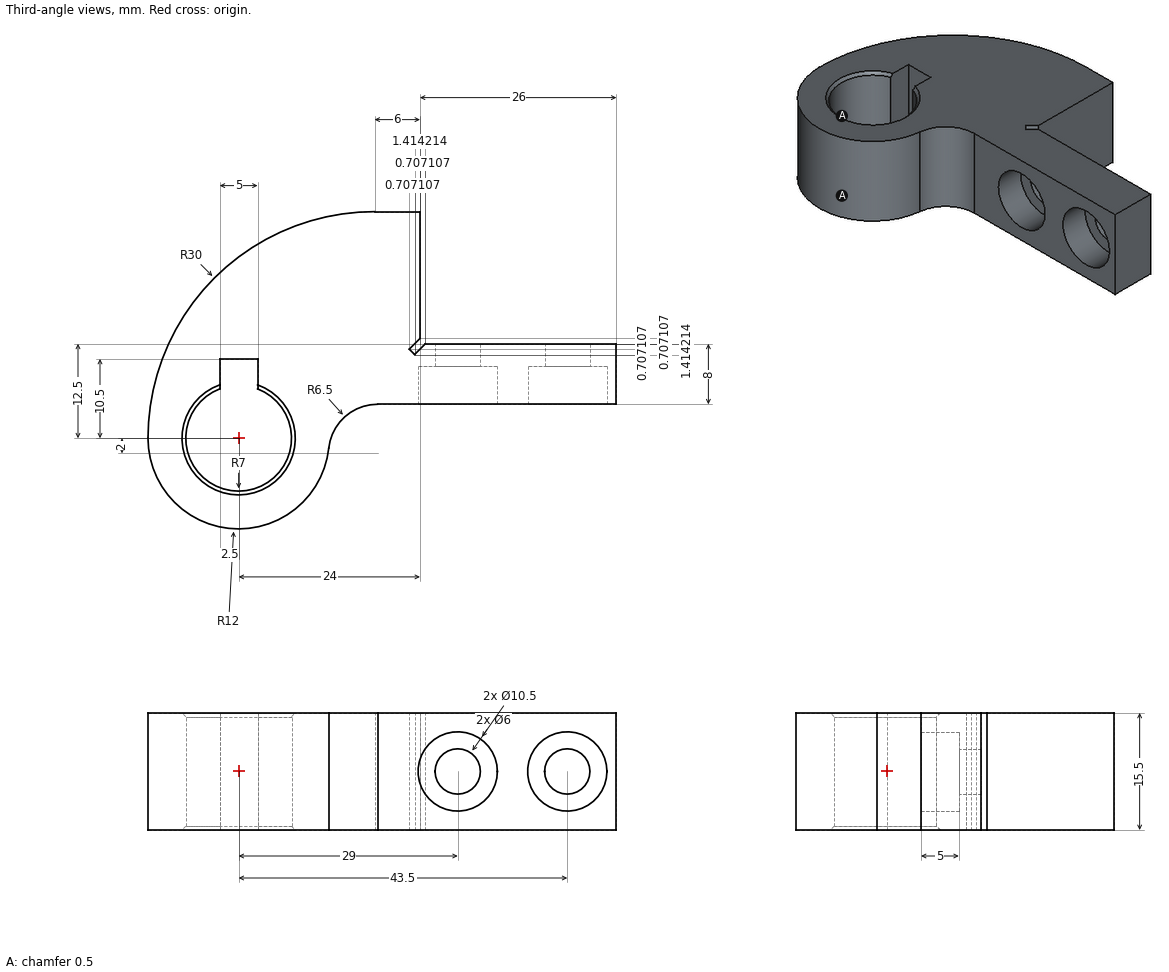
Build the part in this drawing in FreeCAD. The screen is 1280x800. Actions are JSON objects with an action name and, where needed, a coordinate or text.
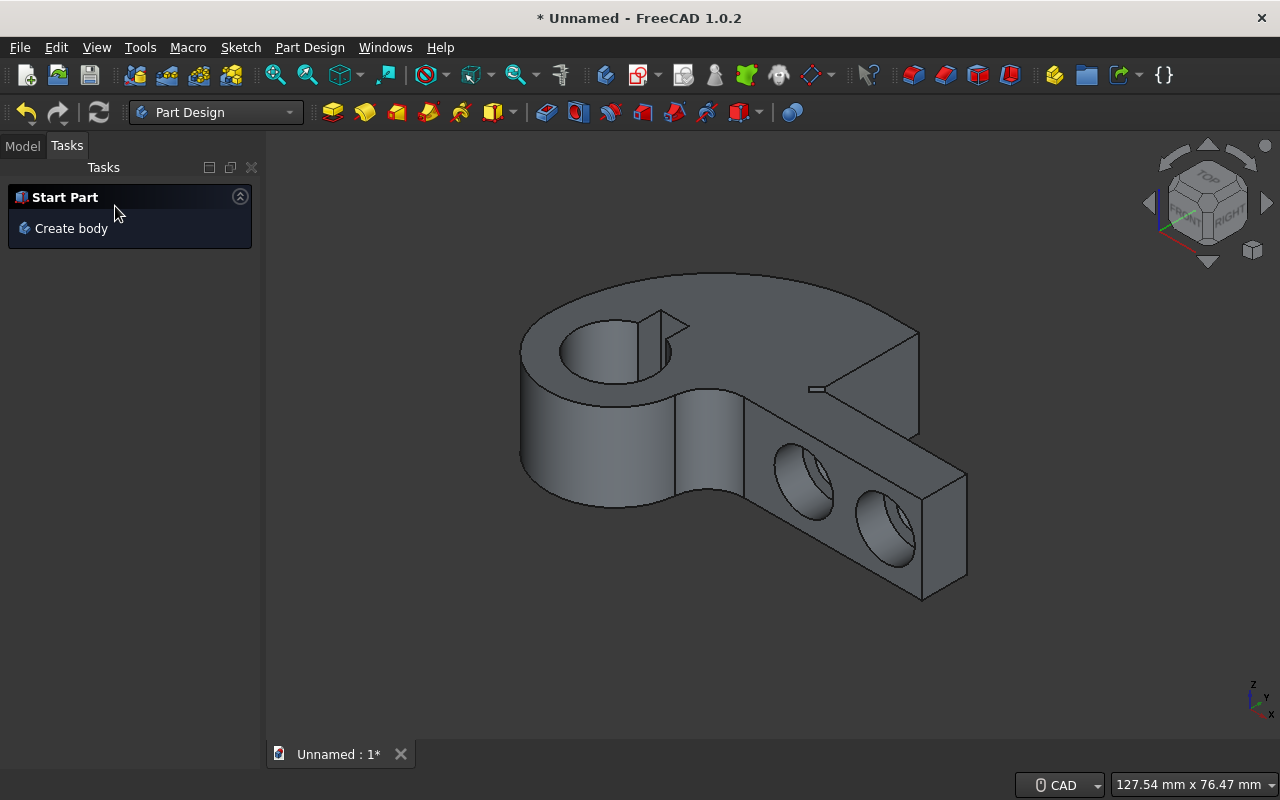
{"action": "left_click", "coordinate": [563, 341]}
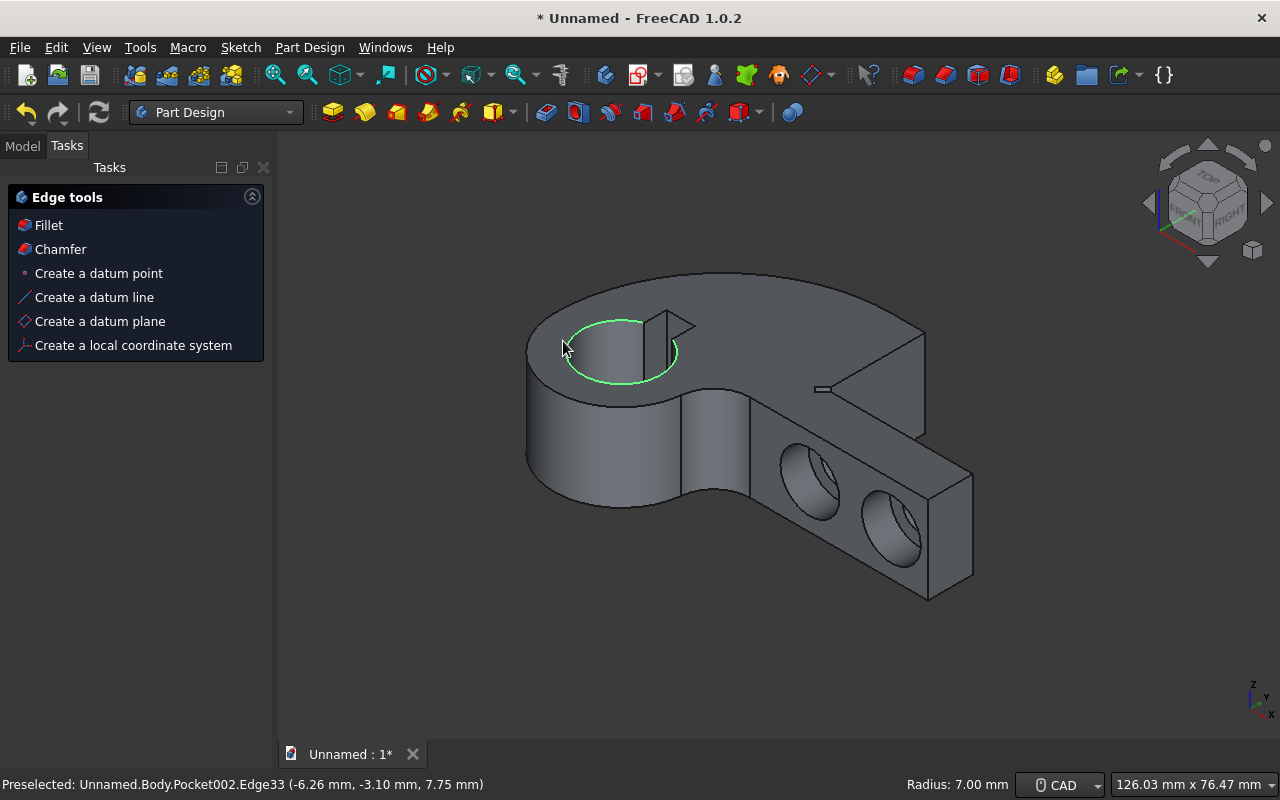
{"action": "key", "text": "2"}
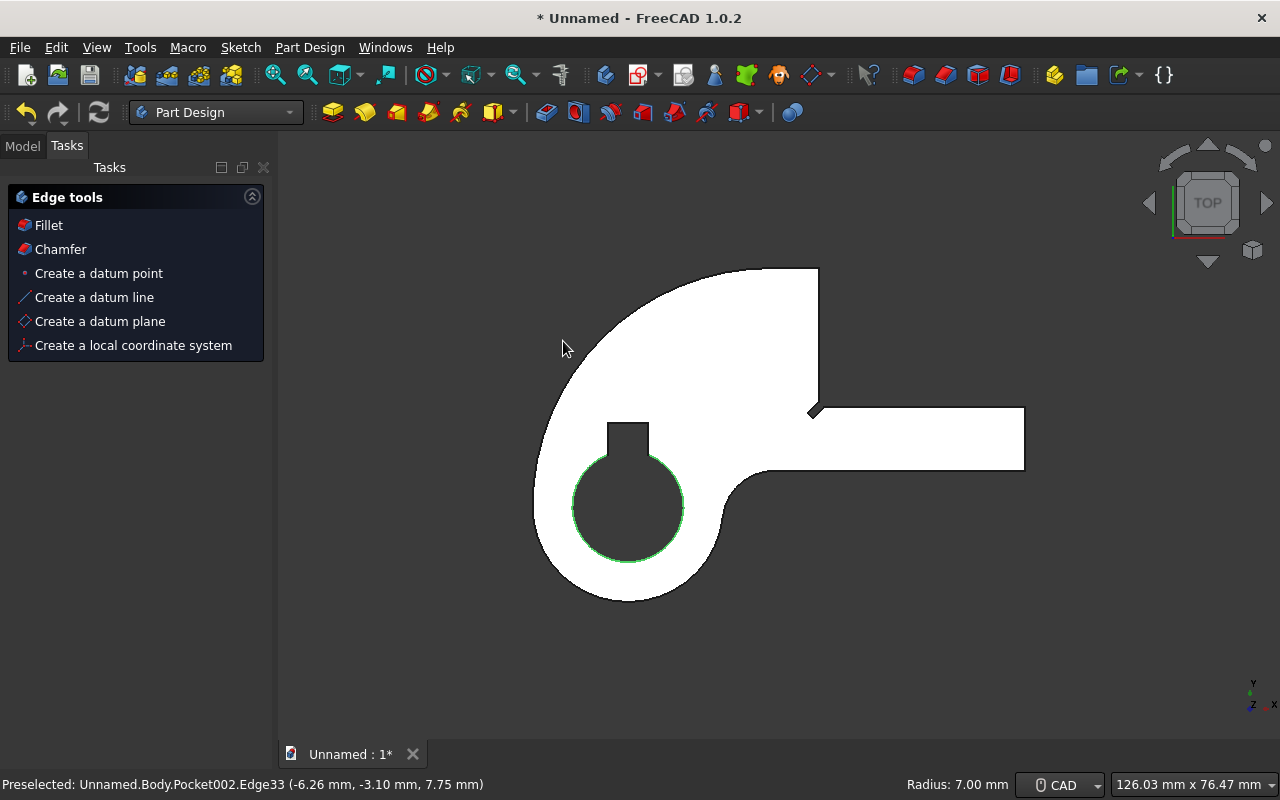
{"action": "key", "text": "0"}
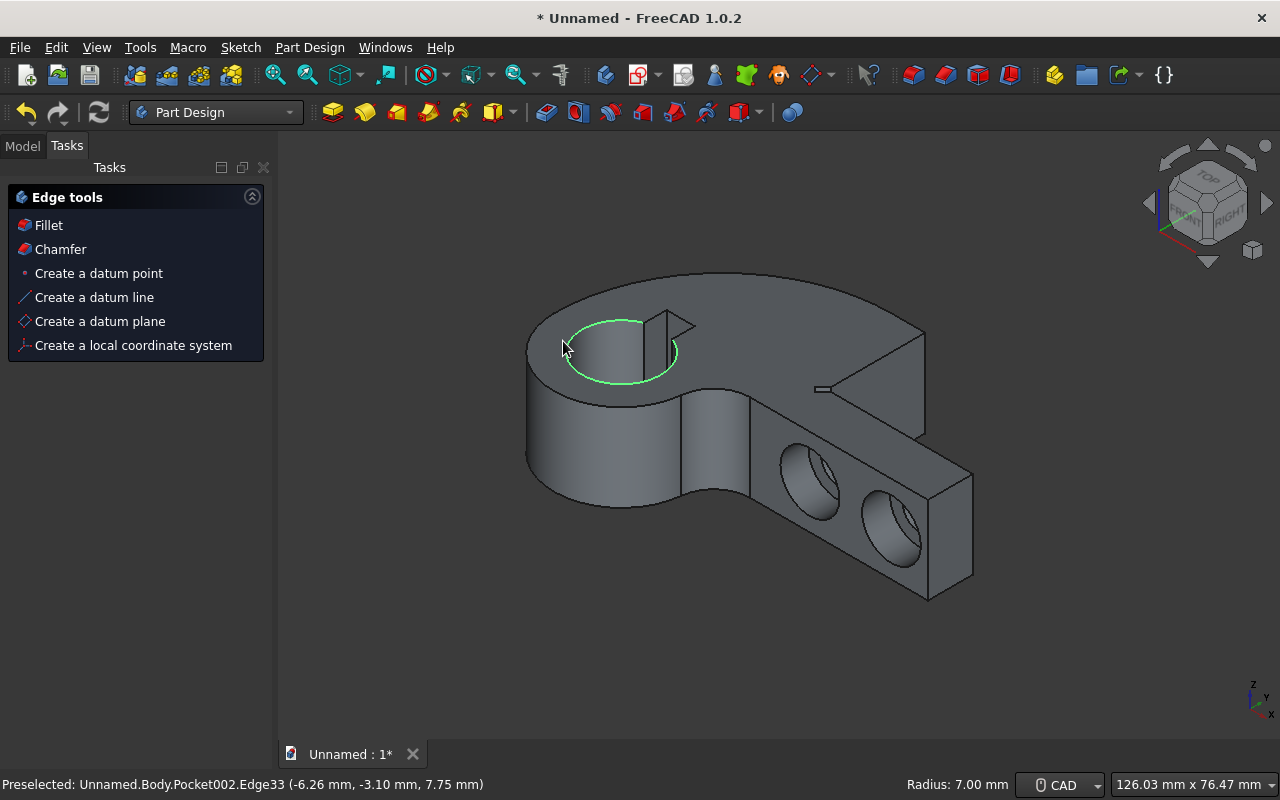
{"action": "key", "text": "1"}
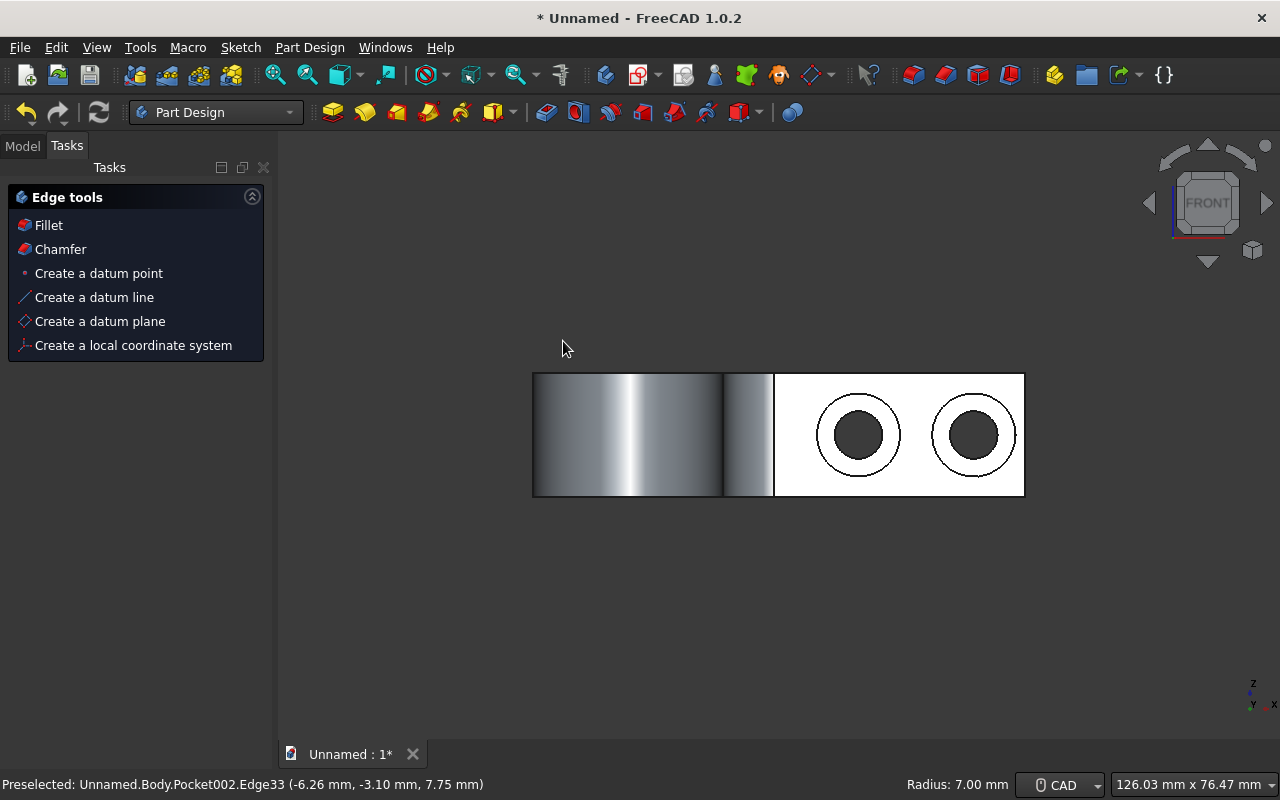
{"action": "key", "text": "3"}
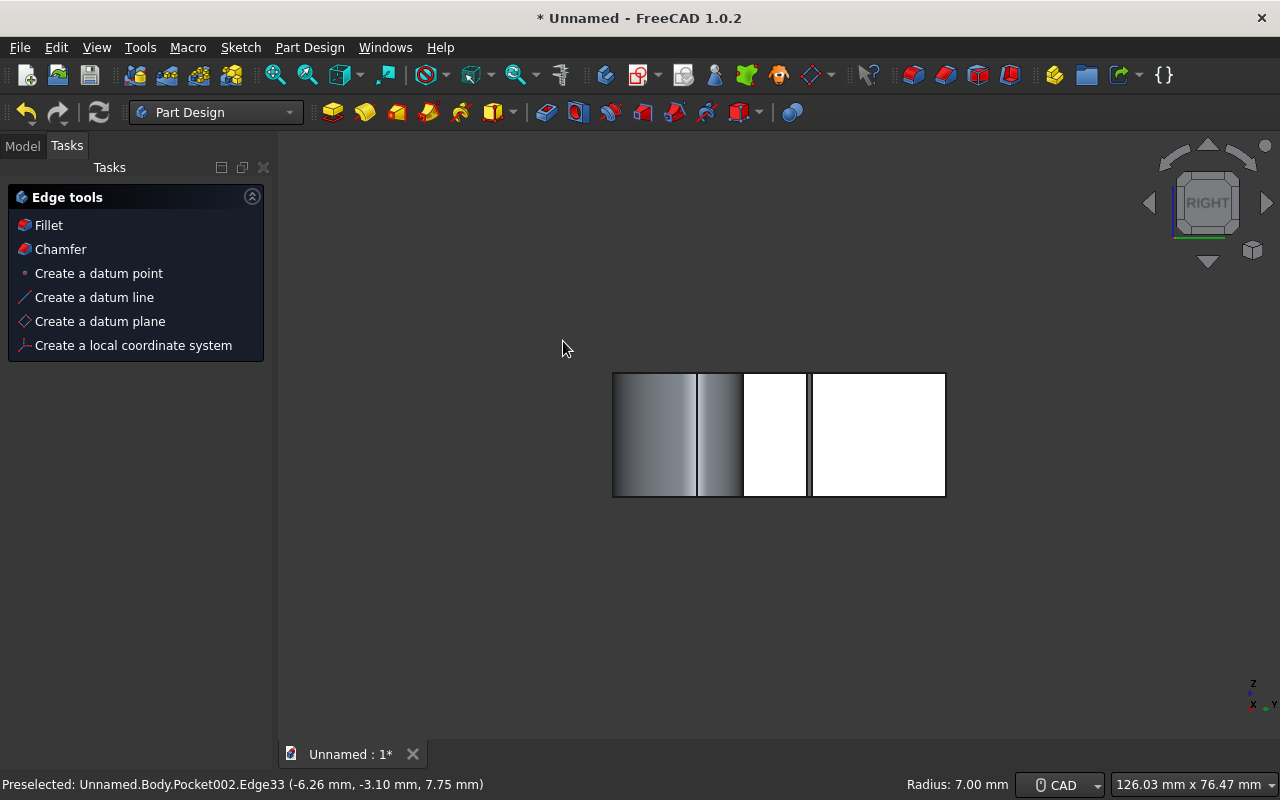
{"action": "left_click", "coordinate": [276, 76]}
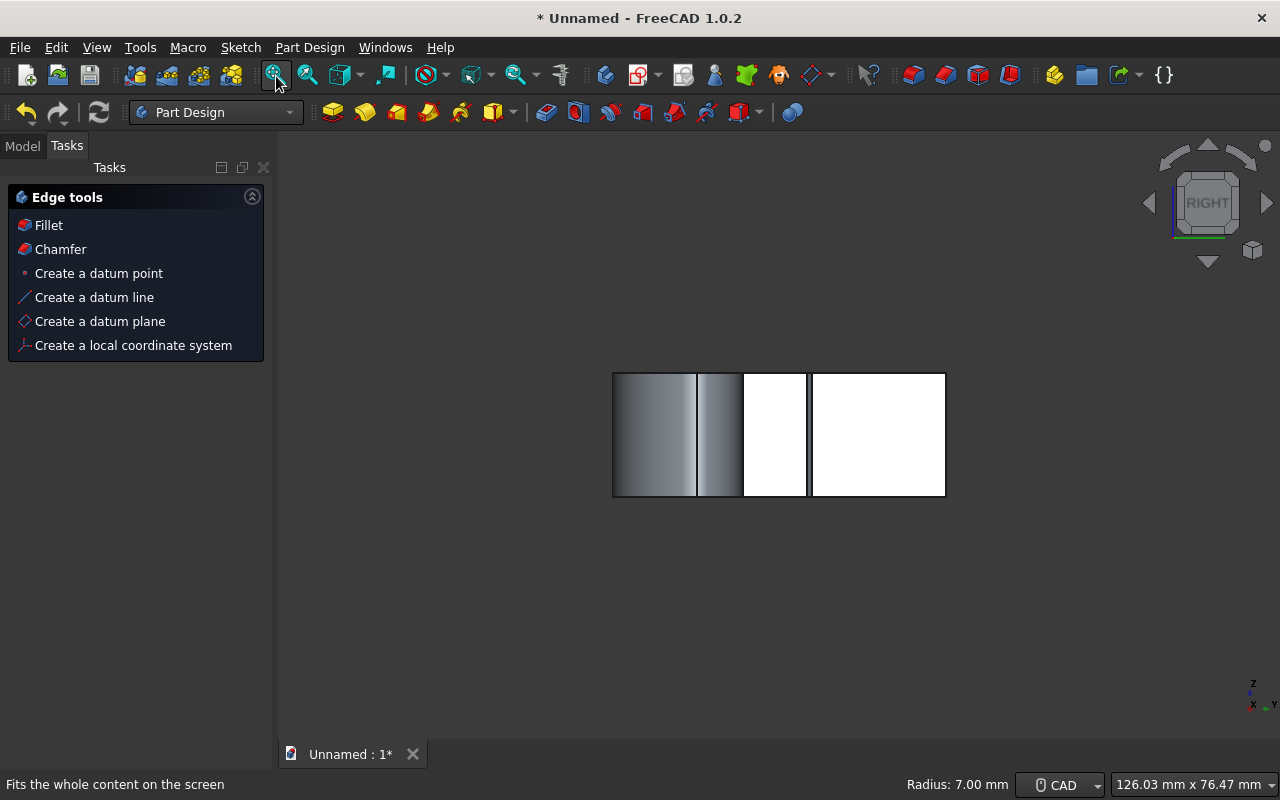
{"action": "key", "text": "5"}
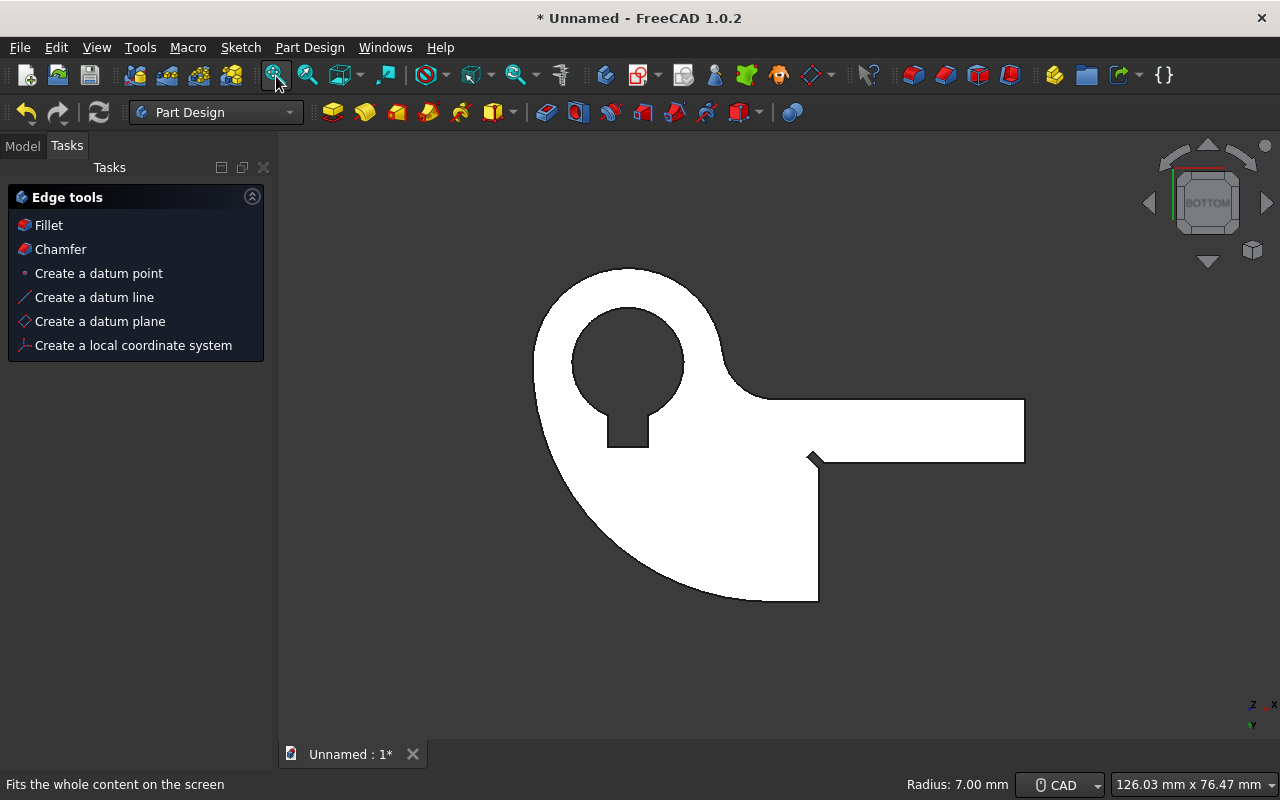
{"action": "left_click", "coordinate": [628, 307], "text": "ctrl"}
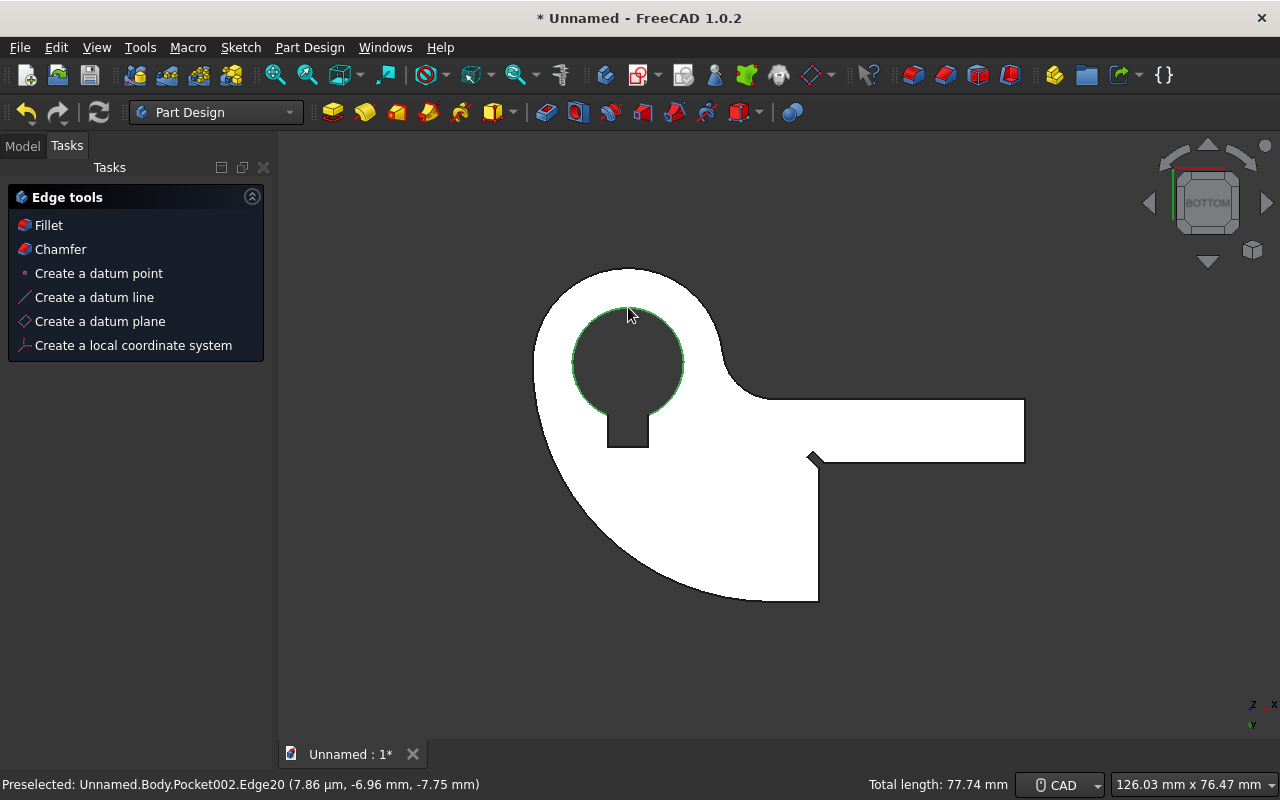
{"action": "left_click", "coordinate": [946, 76]}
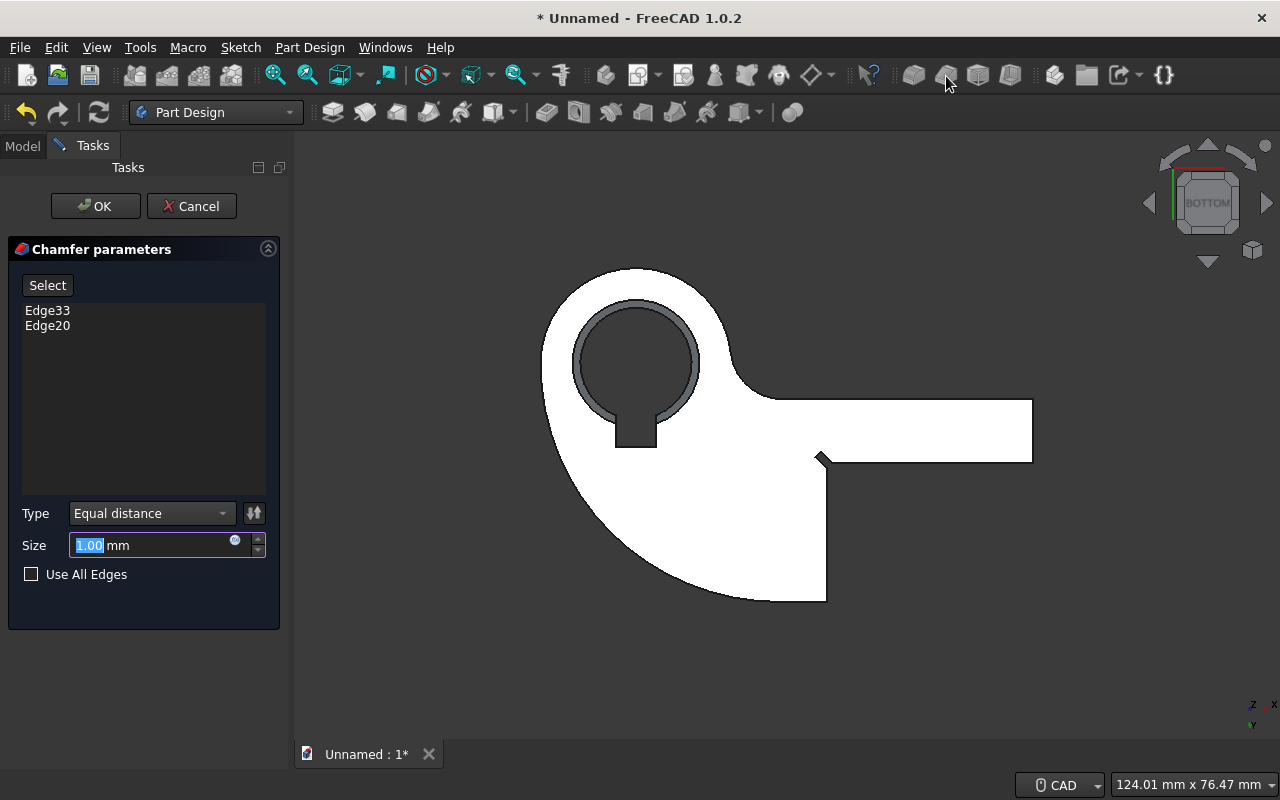
{"action": "type", "text": "0.5"}
{"action": "key", "text": "Tab"}